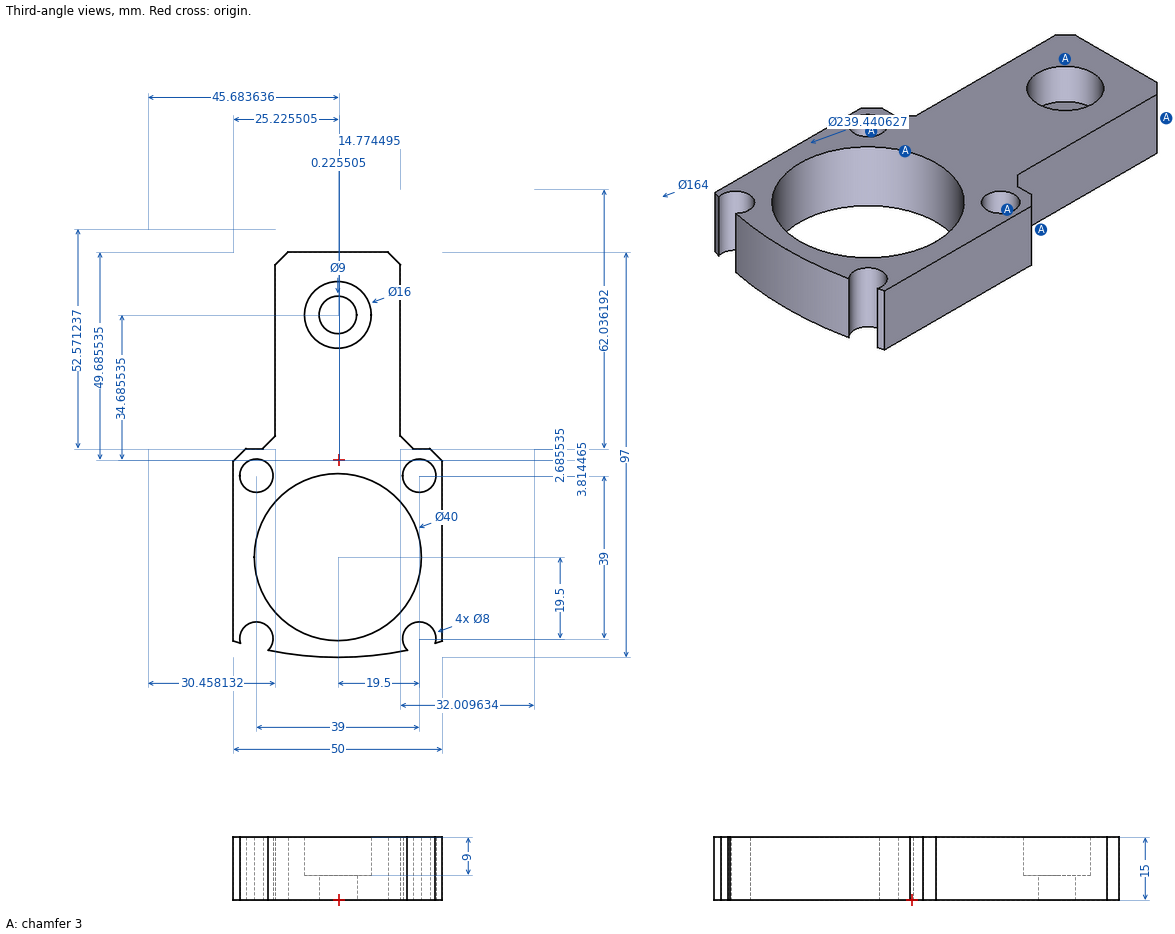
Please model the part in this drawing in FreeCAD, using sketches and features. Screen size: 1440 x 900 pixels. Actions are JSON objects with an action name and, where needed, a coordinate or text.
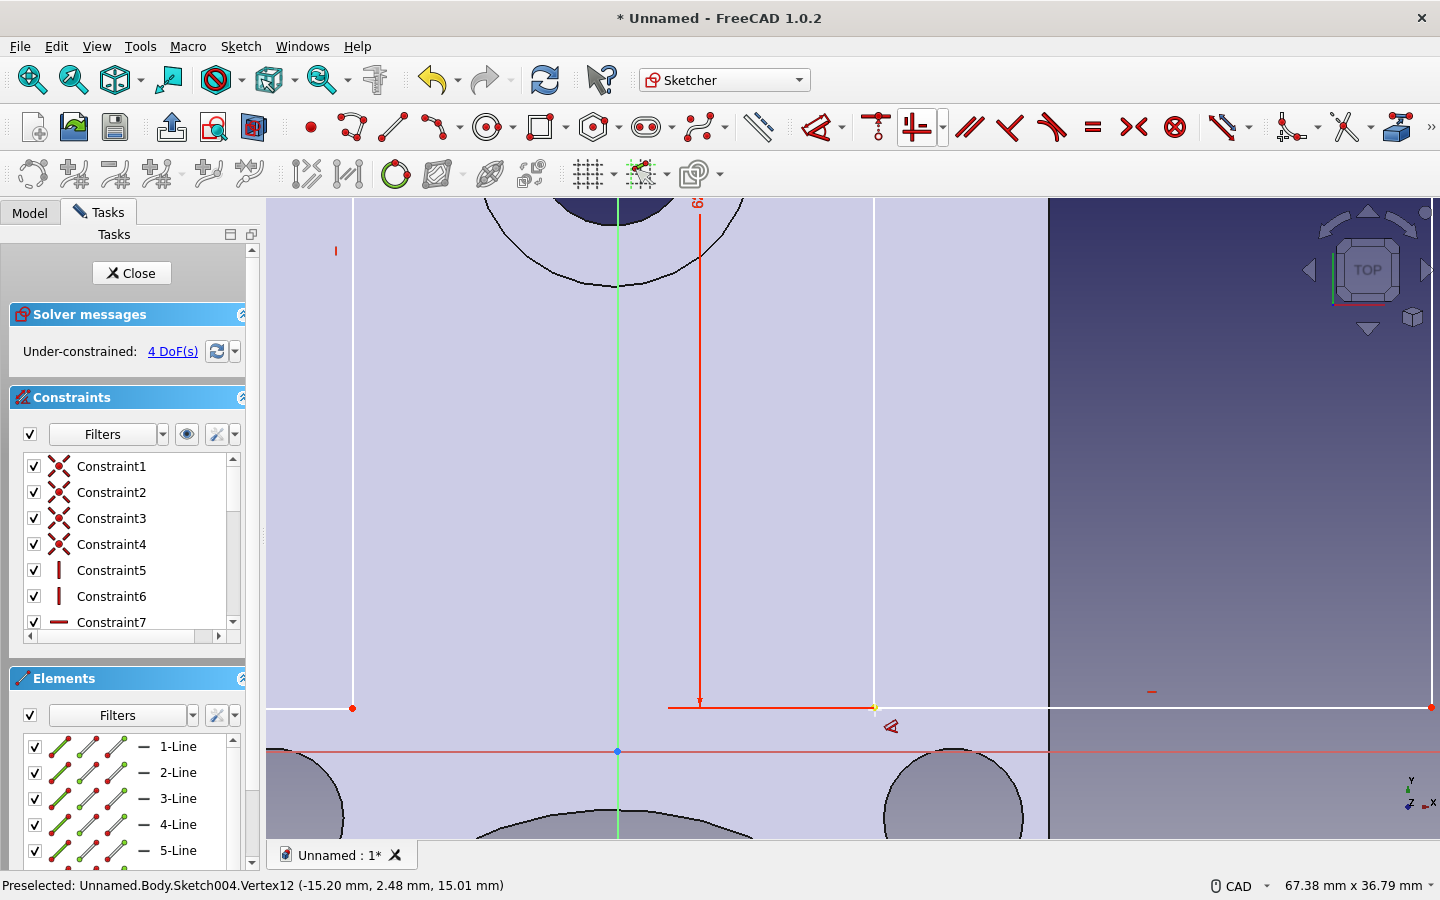
{"action": "left_click", "coordinate": [874, 708]}
{"action": "left_click", "coordinate": [908, 730]}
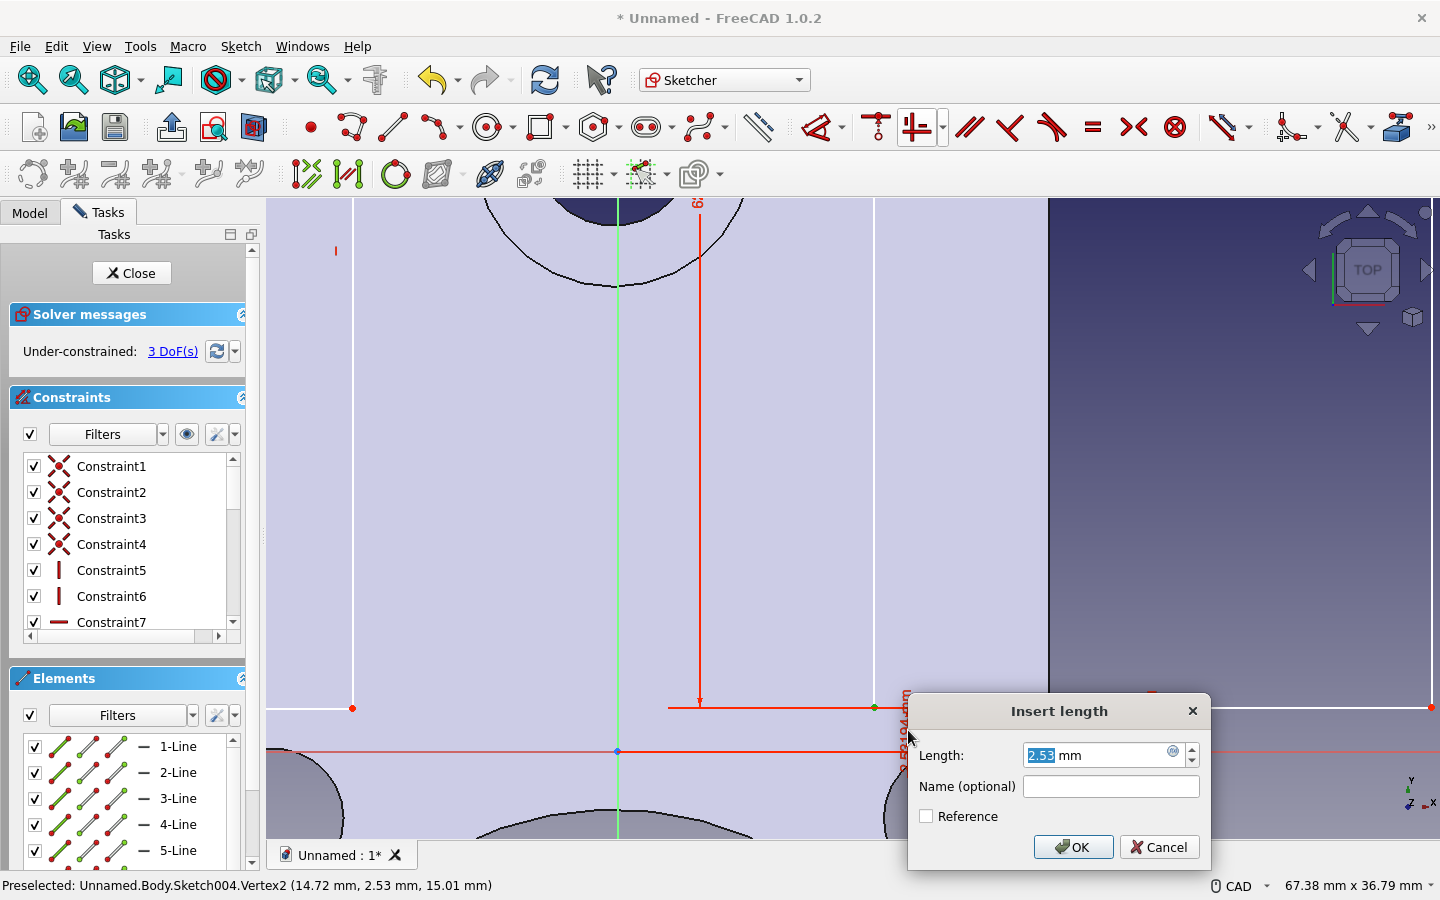
{"action": "type", "text": "2.685535"}
{"action": "key", "text": "Return"}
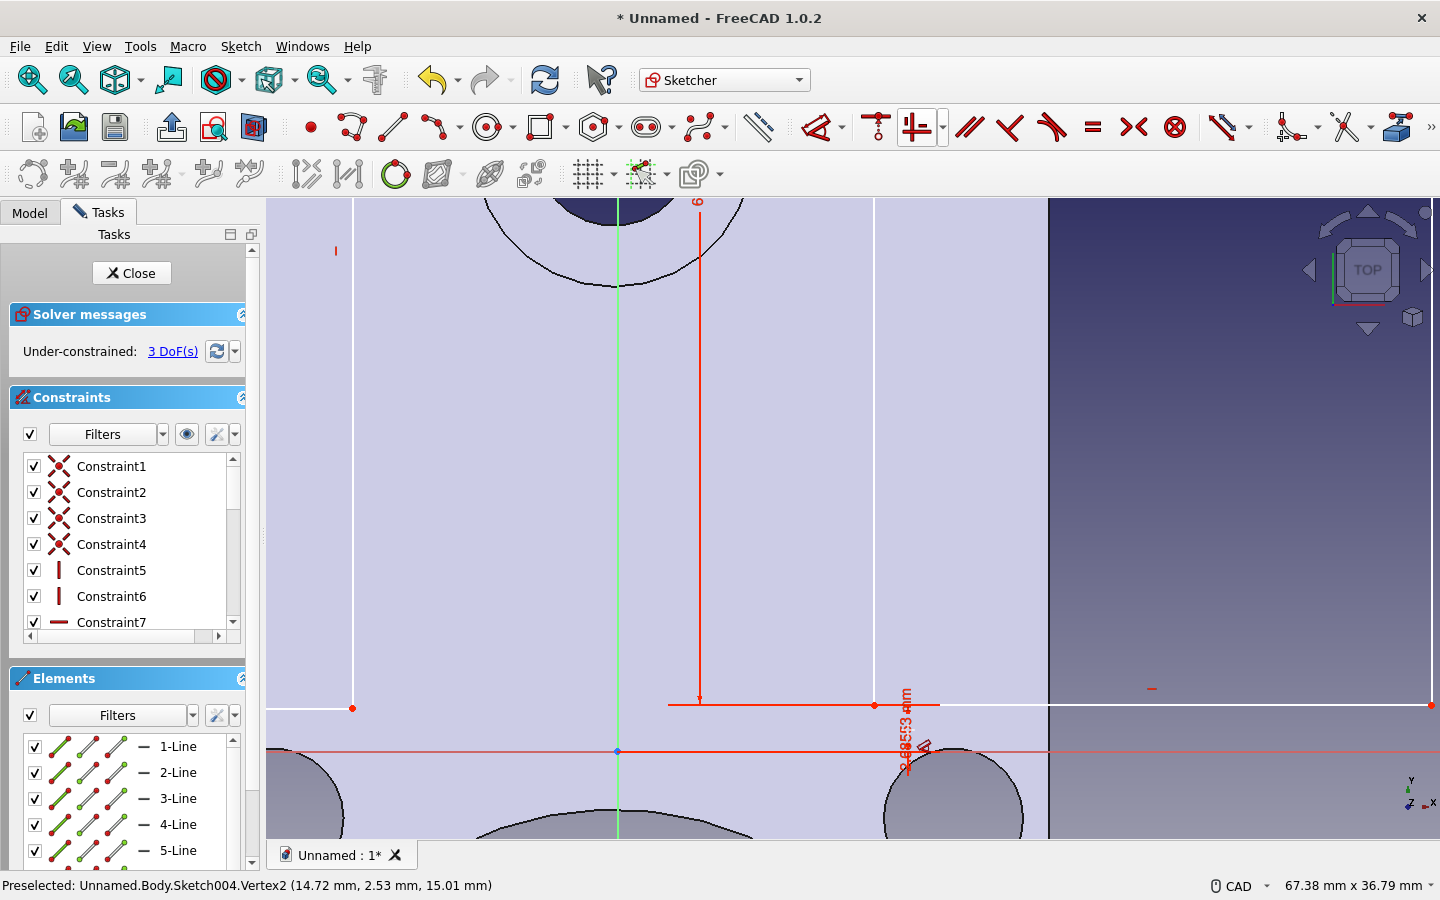
{"action": "scroll", "coordinate": [876, 711], "scroll_direction": "down", "scroll_amount": 5}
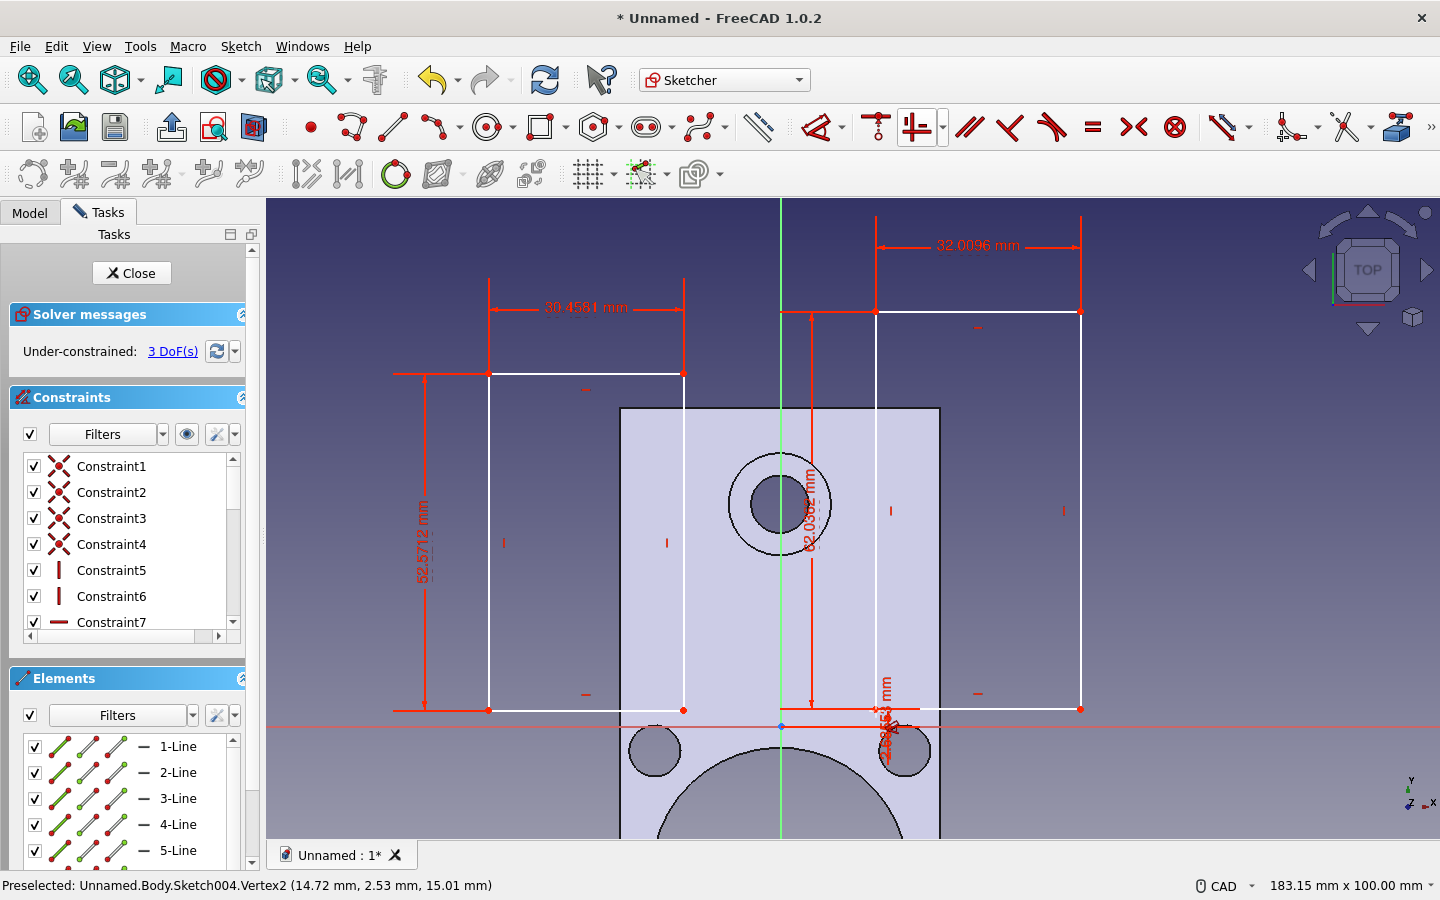
{"action": "scroll", "coordinate": [489, 711], "scroll_direction": "up", "scroll_amount": 5}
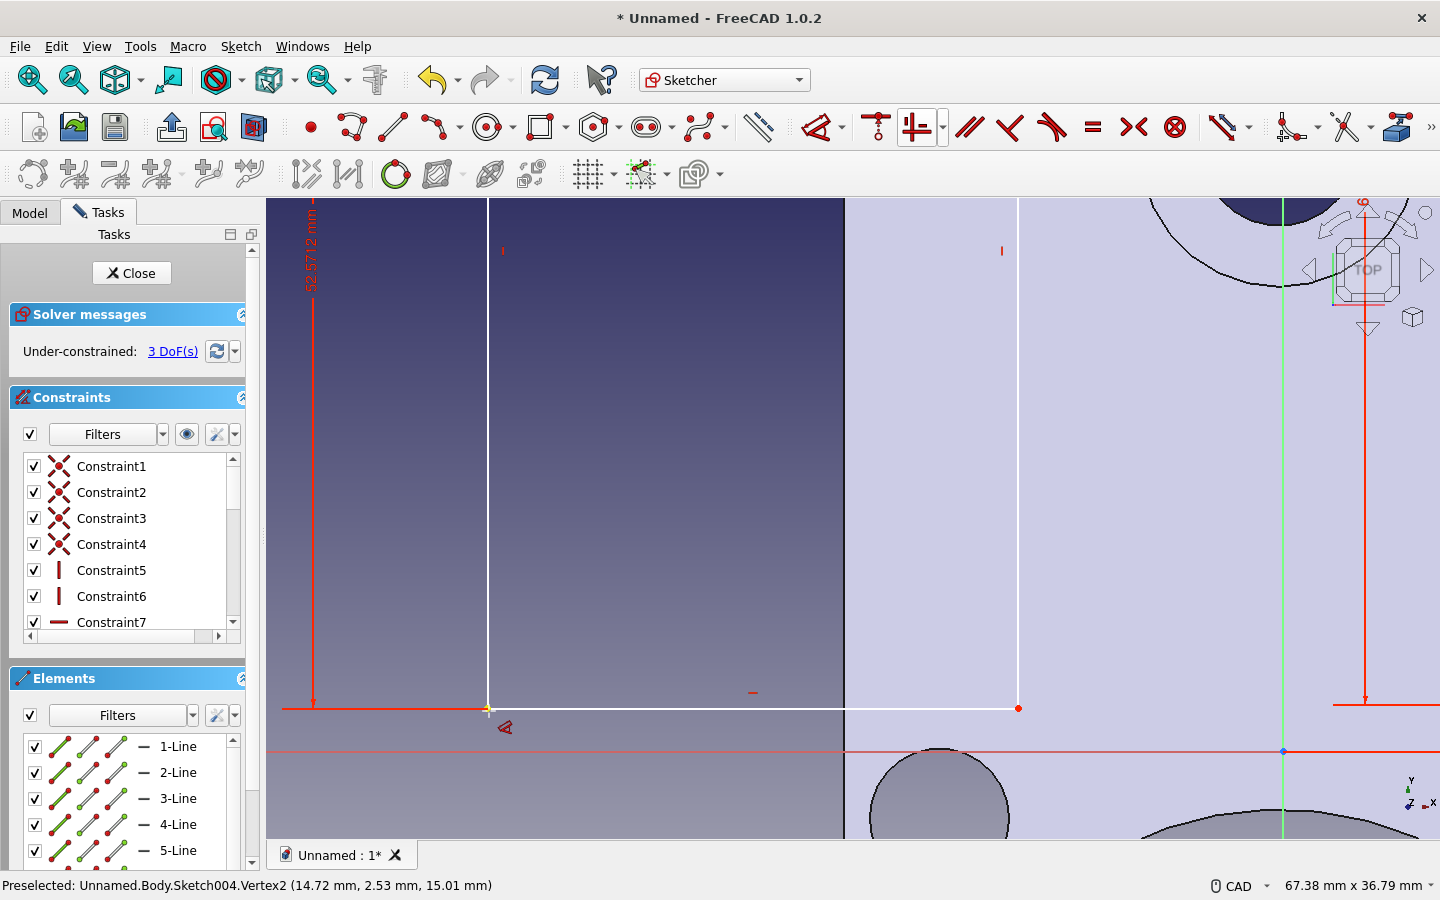
{"action": "left_click", "coordinate": [488, 709]}
{"action": "left_click", "coordinate": [454, 730]}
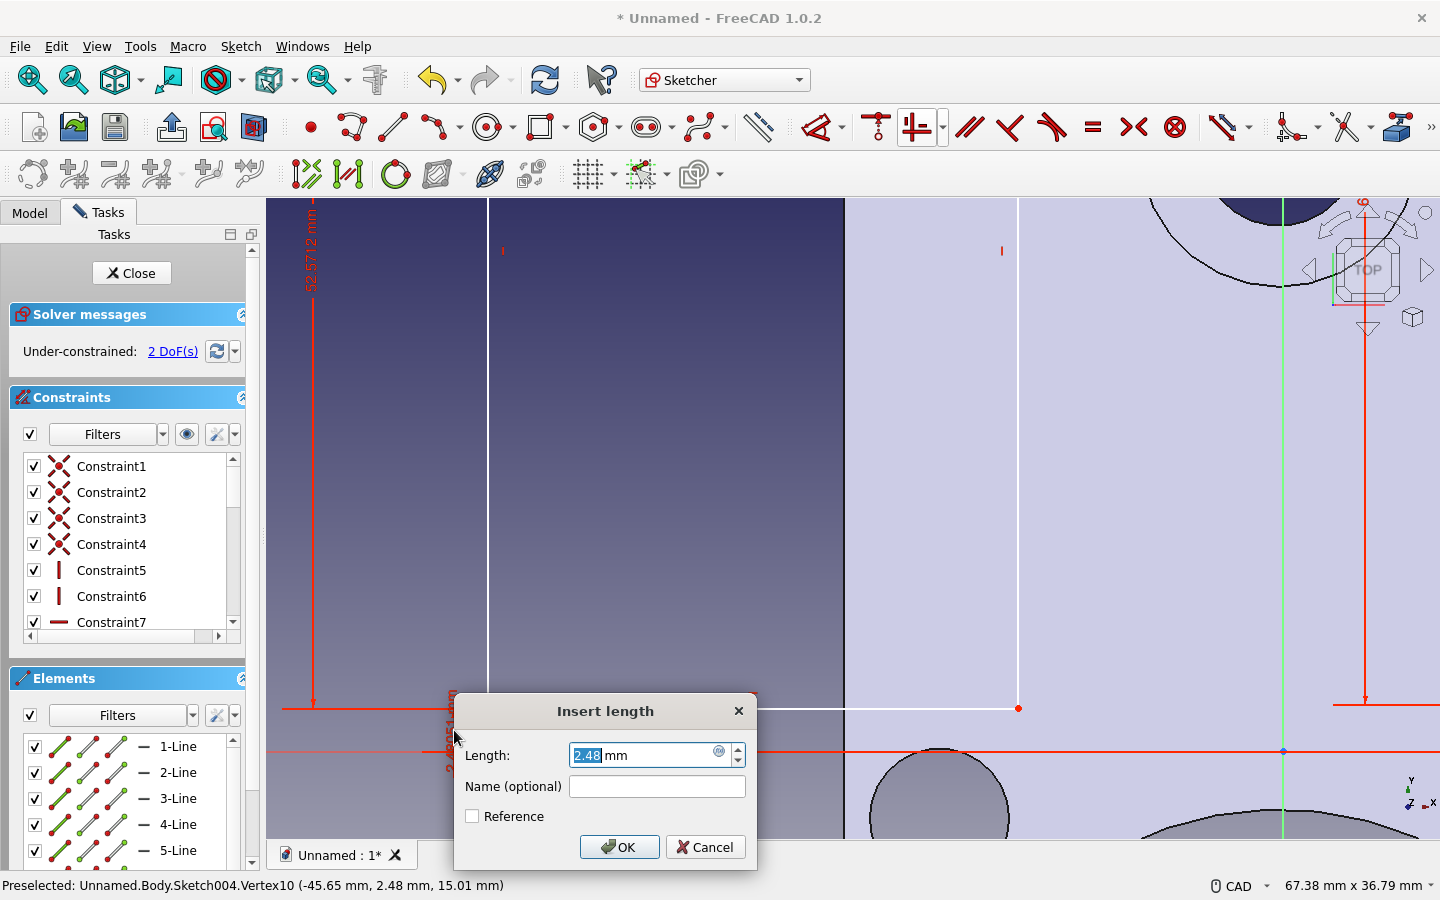
{"action": "type", "text": "2.685535"}
{"action": "key", "text": "Return"}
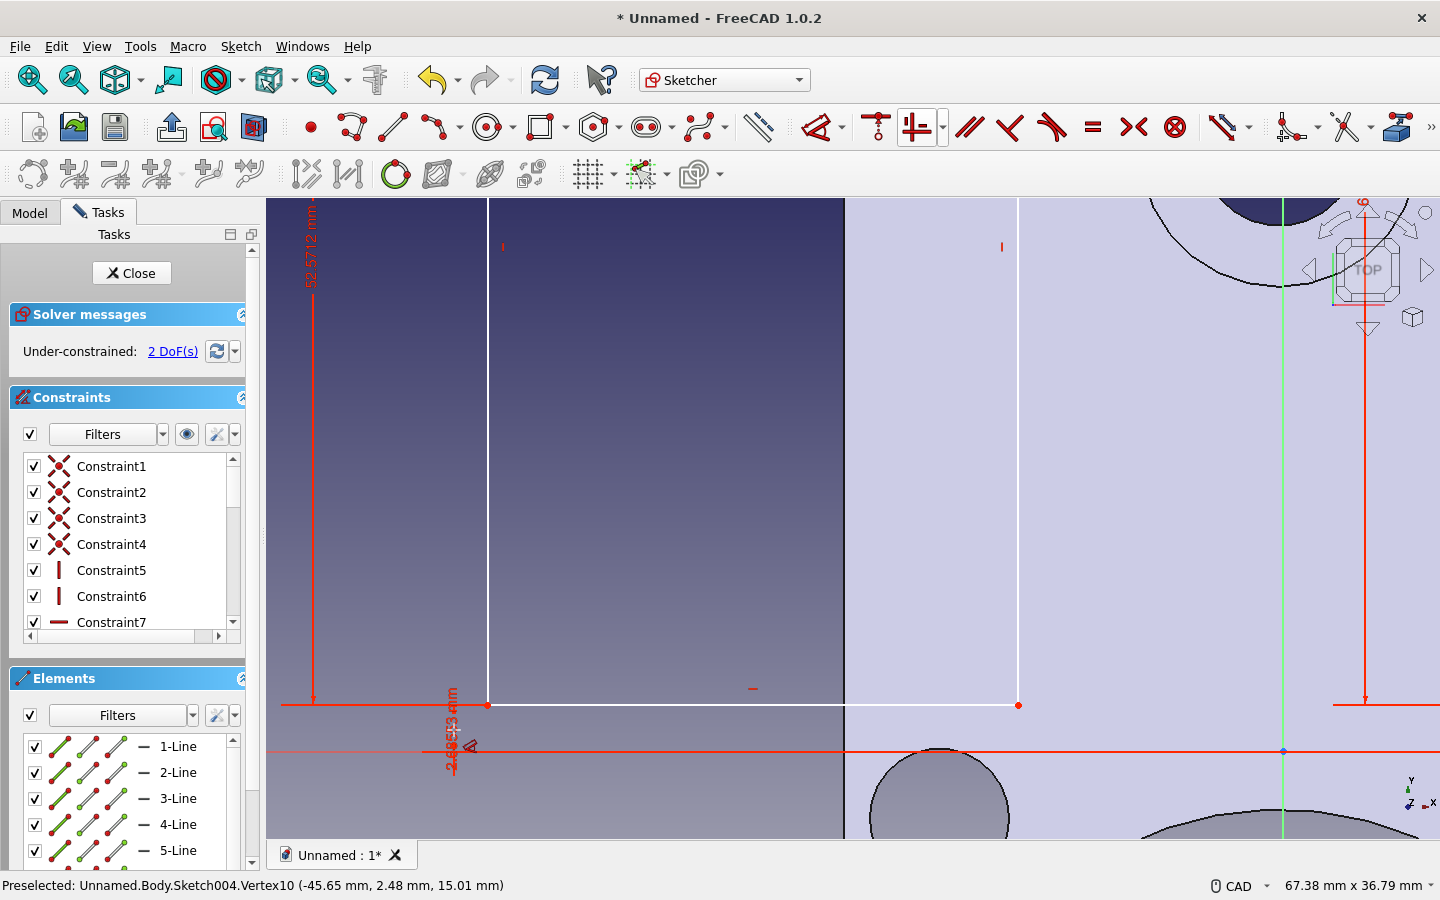
{"action": "scroll", "coordinate": [489, 711], "scroll_direction": "down", "scroll_amount": 5}